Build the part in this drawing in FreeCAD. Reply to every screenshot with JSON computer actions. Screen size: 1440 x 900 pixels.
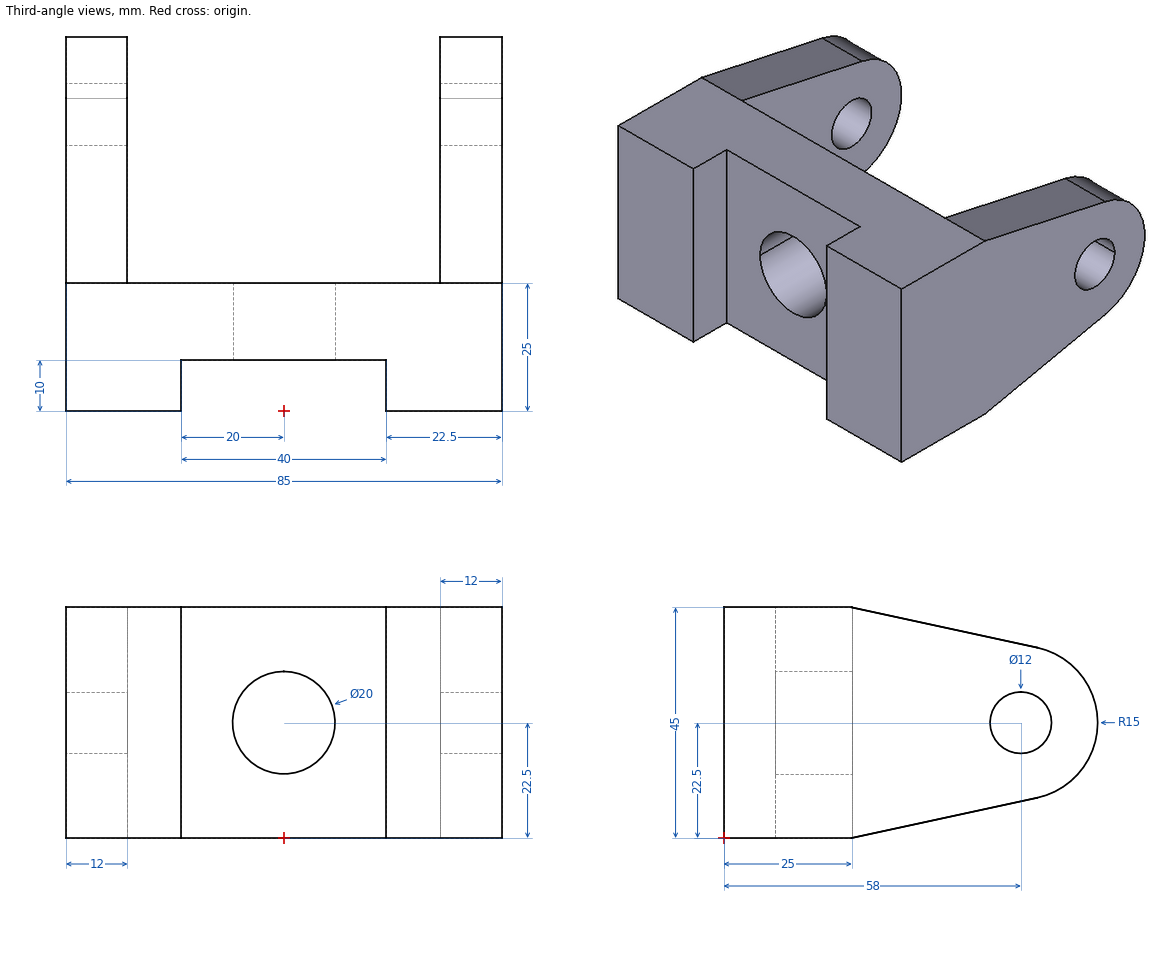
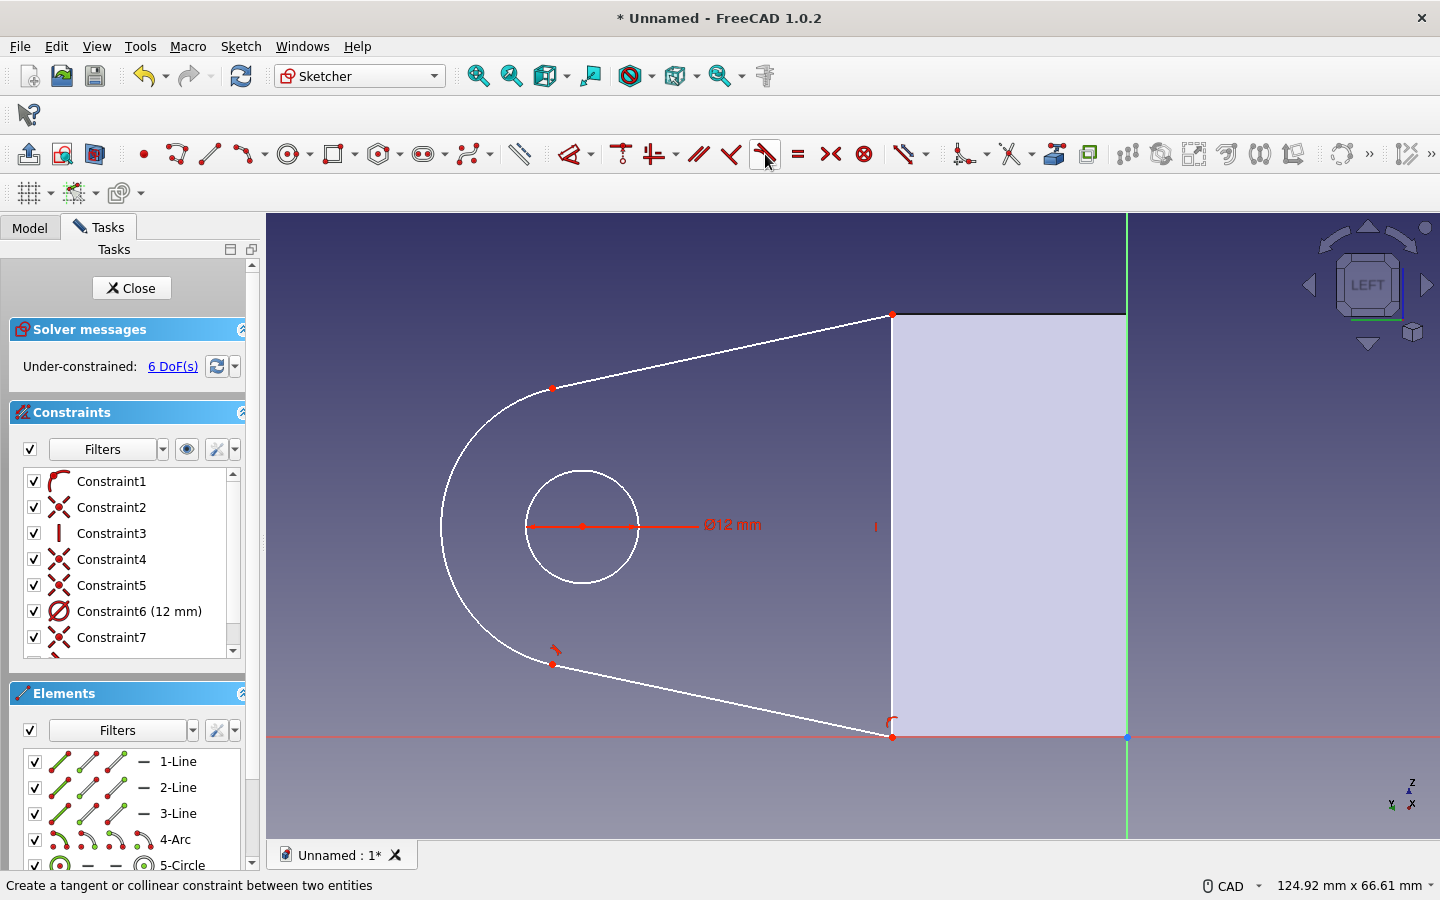
{"action": "left_click", "coordinate": [790, 337]}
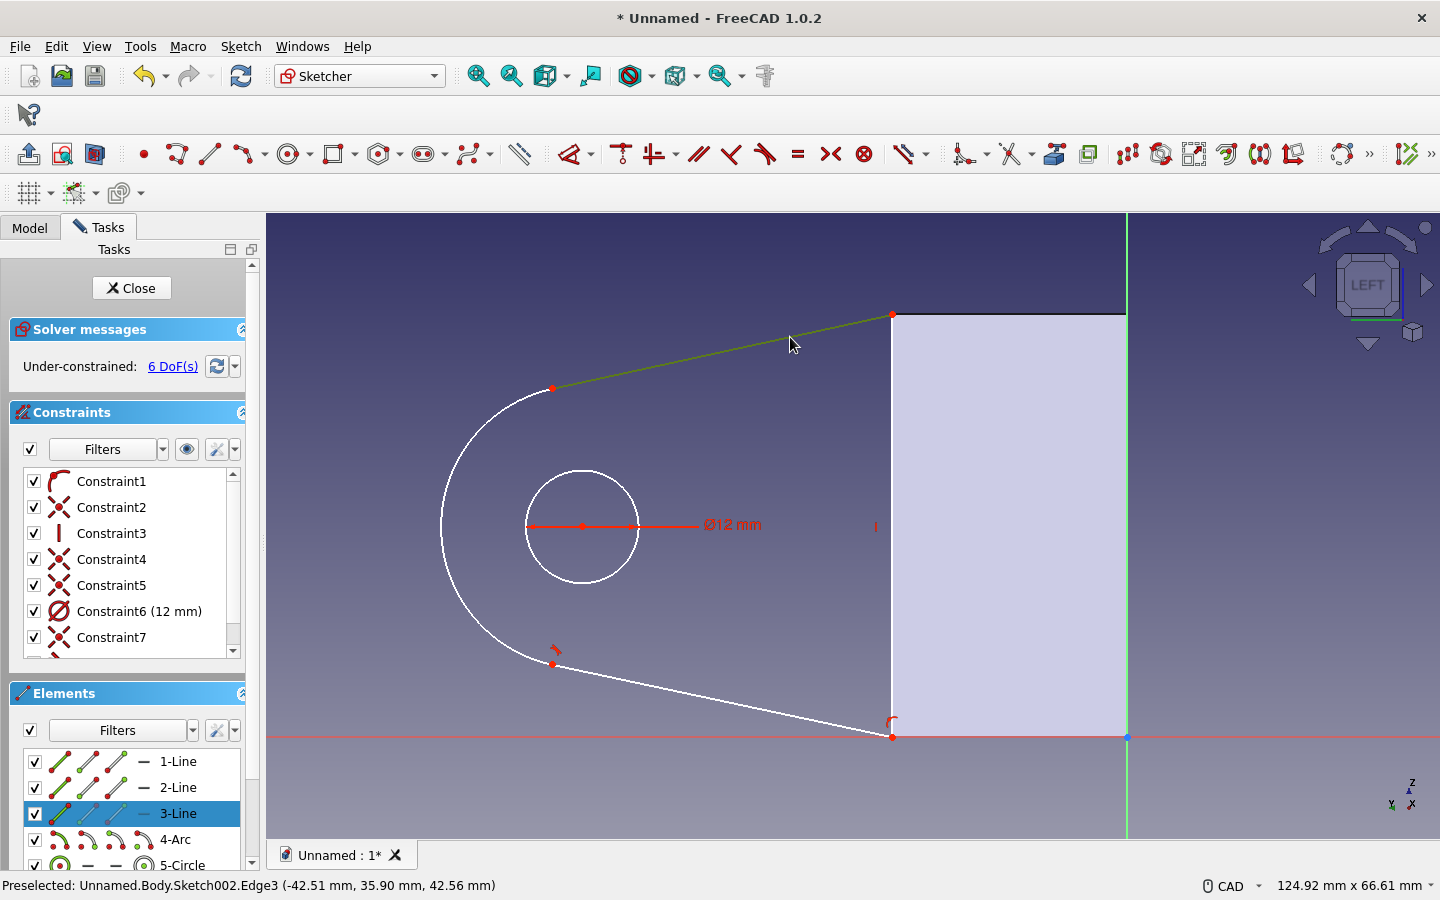
{"action": "left_click", "coordinate": [461, 454]}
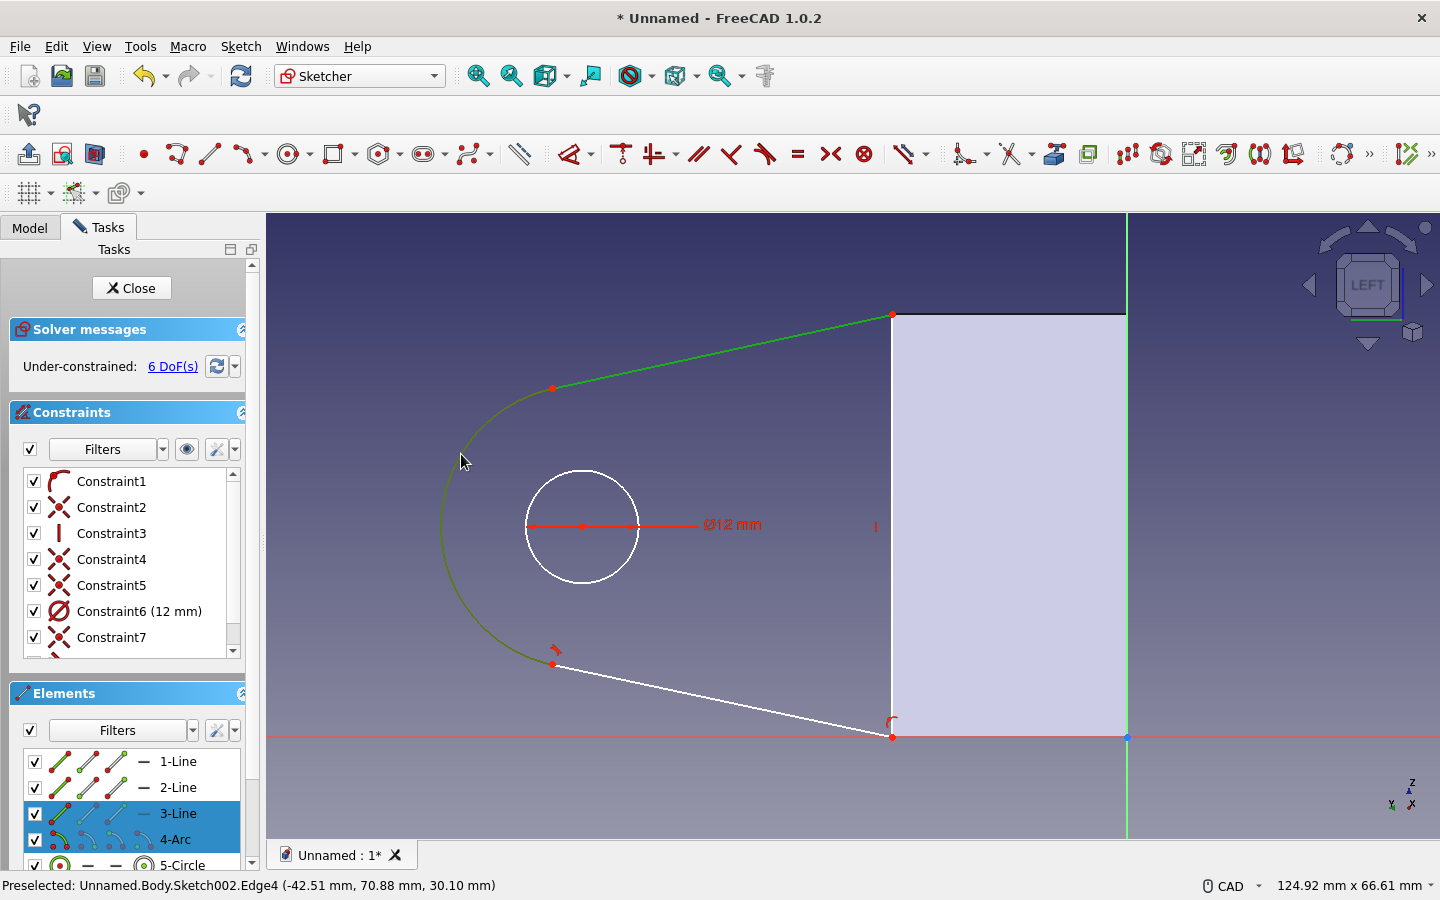
{"action": "left_click", "coordinate": [765, 154]}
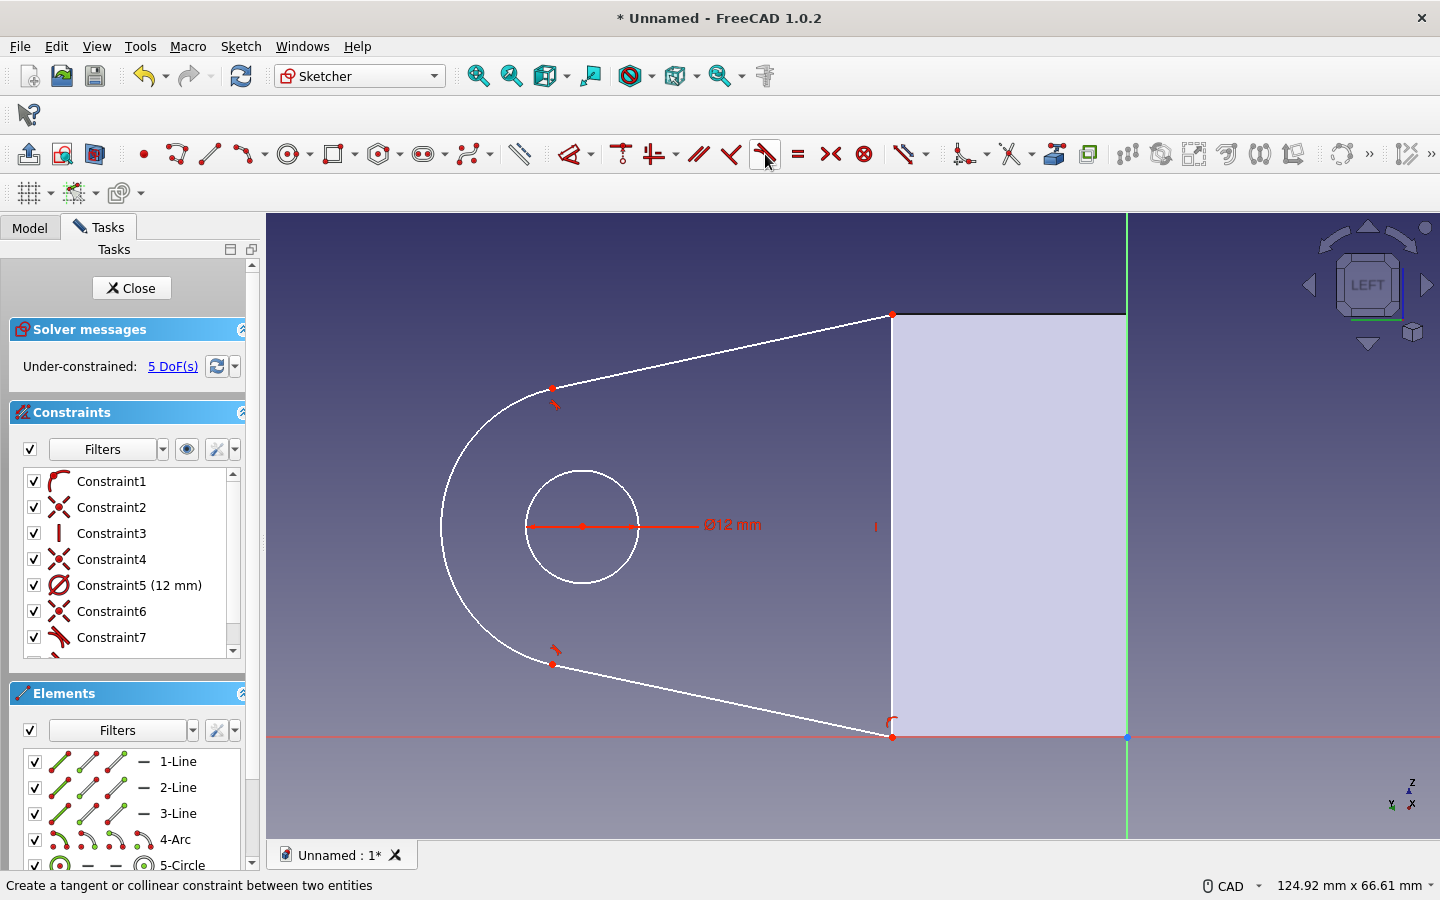
{"action": "key", "text": "d"}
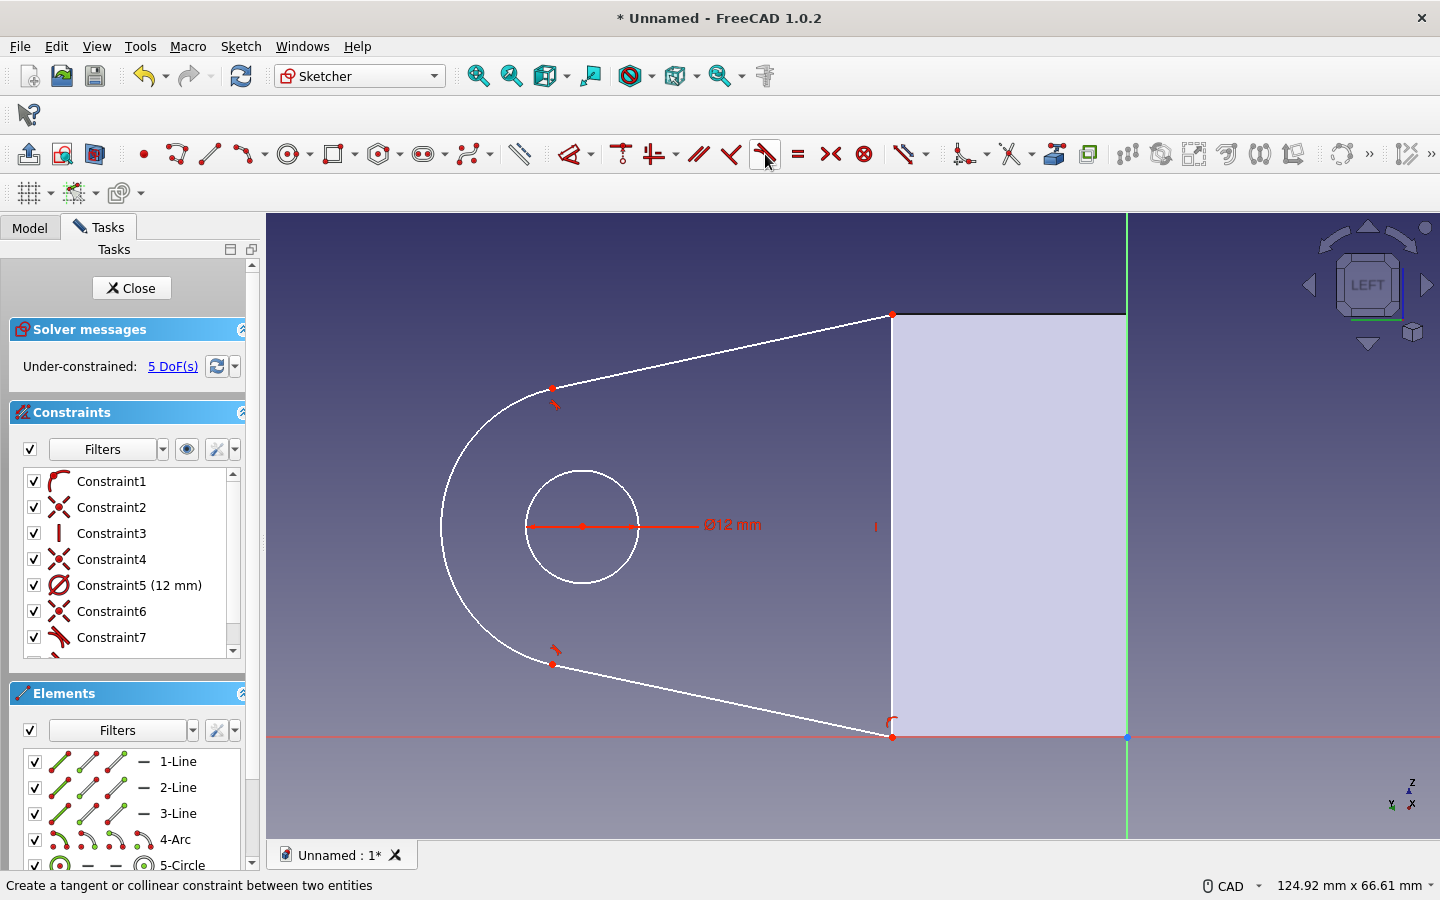
{"action": "left_click", "coordinate": [461, 454]}
{"action": "left_click", "coordinate": [434, 438]}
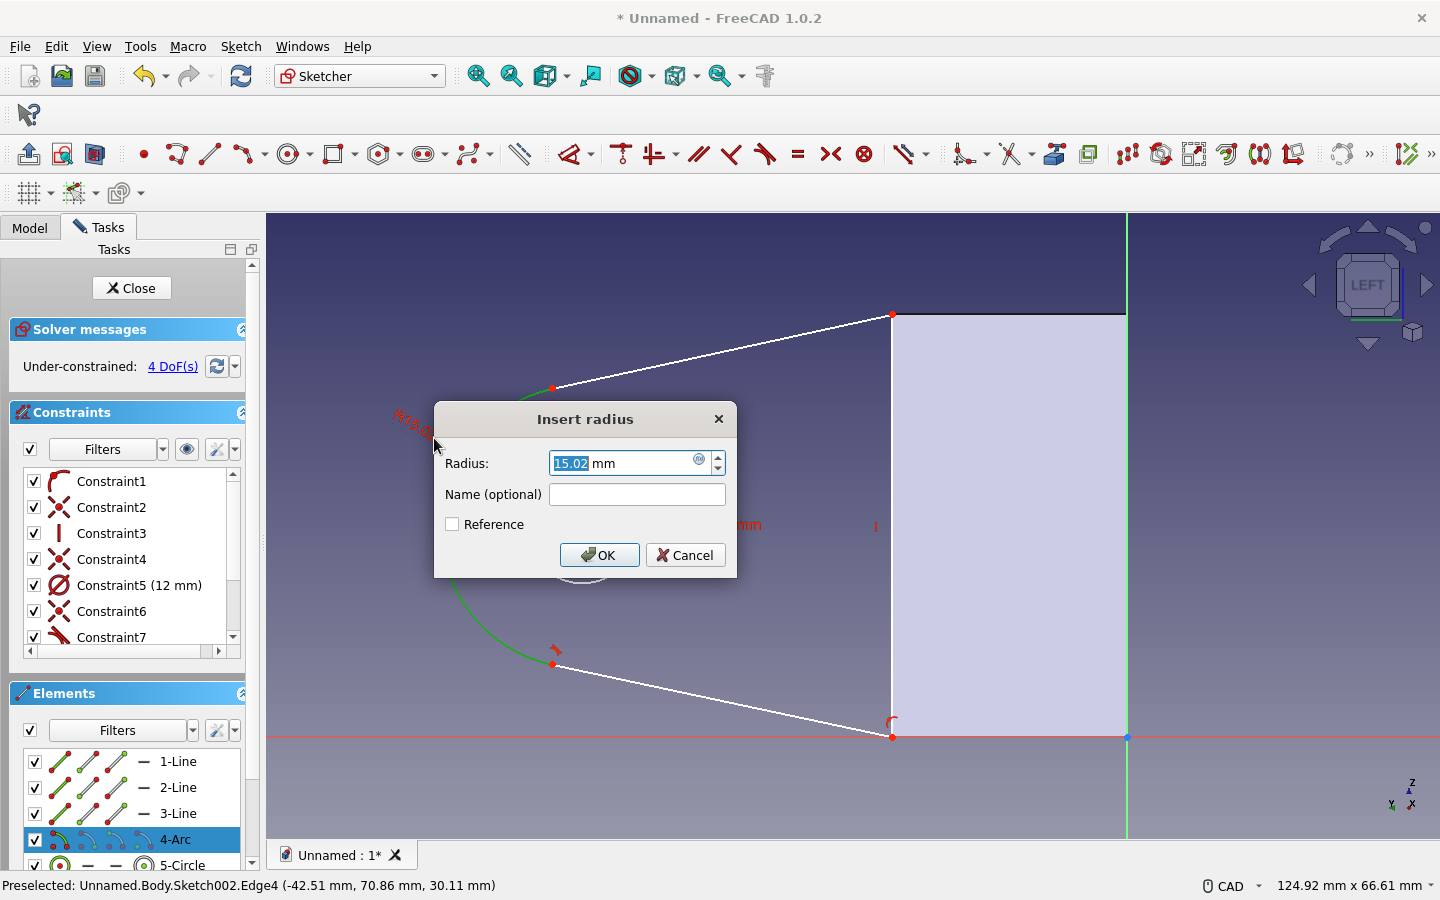
{"action": "type", "text": "15"}
{"action": "key", "text": "Return"}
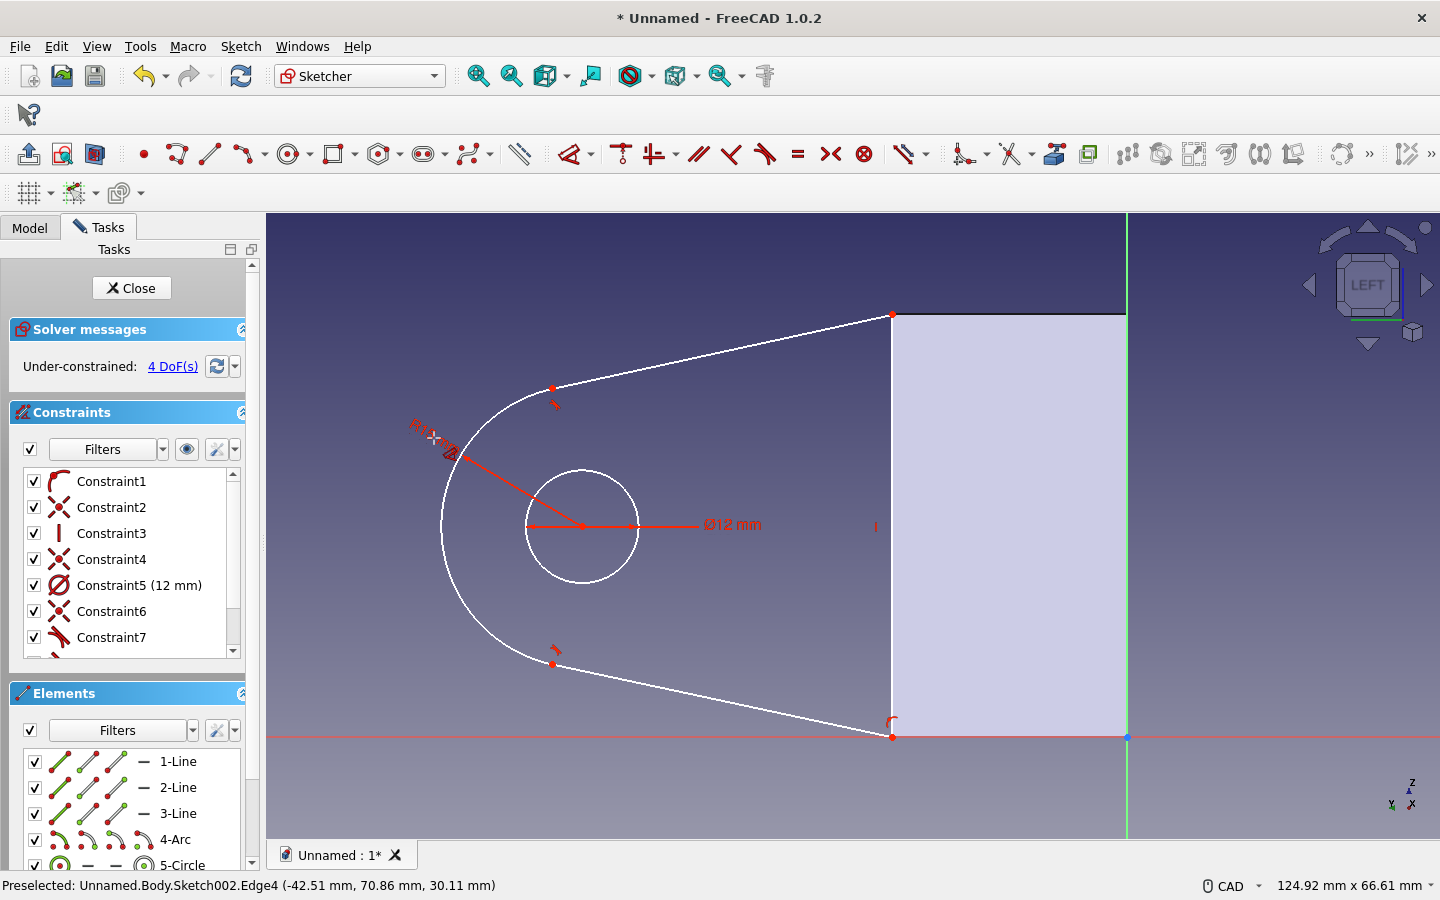
{"action": "left_click", "coordinate": [892, 611]}
{"action": "left_click", "coordinate": [926, 526]}